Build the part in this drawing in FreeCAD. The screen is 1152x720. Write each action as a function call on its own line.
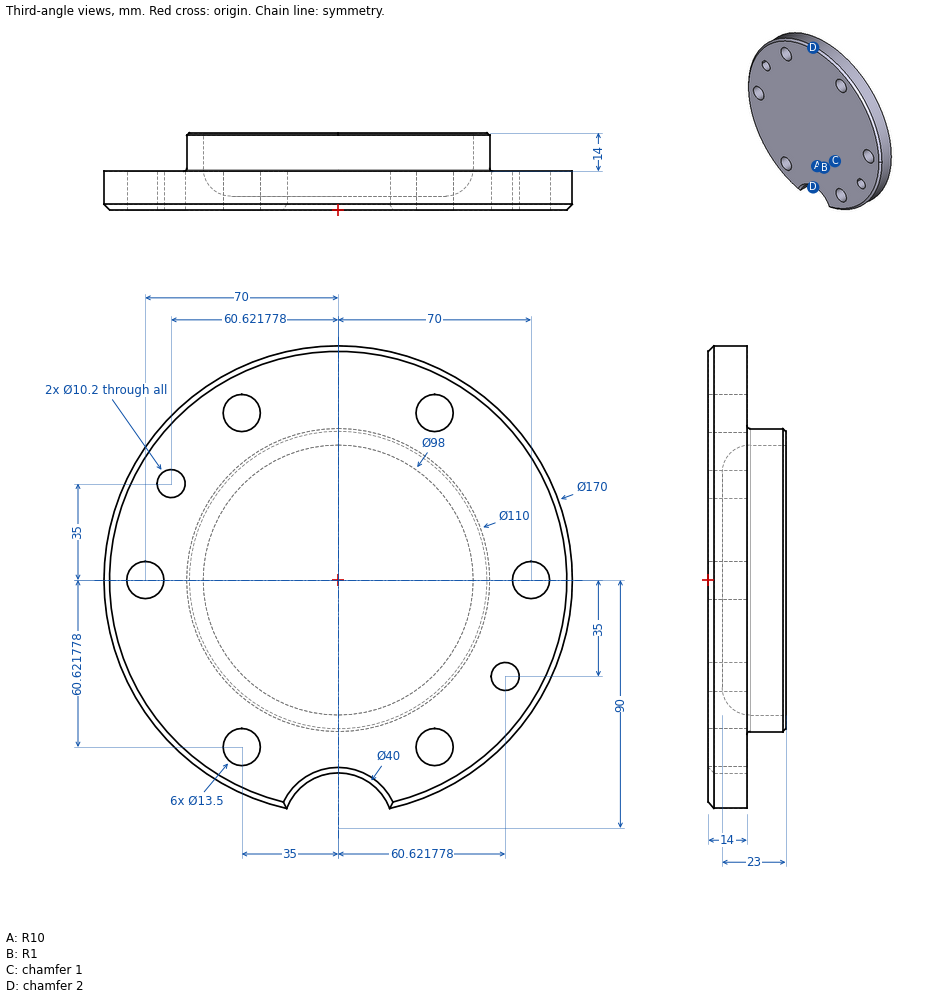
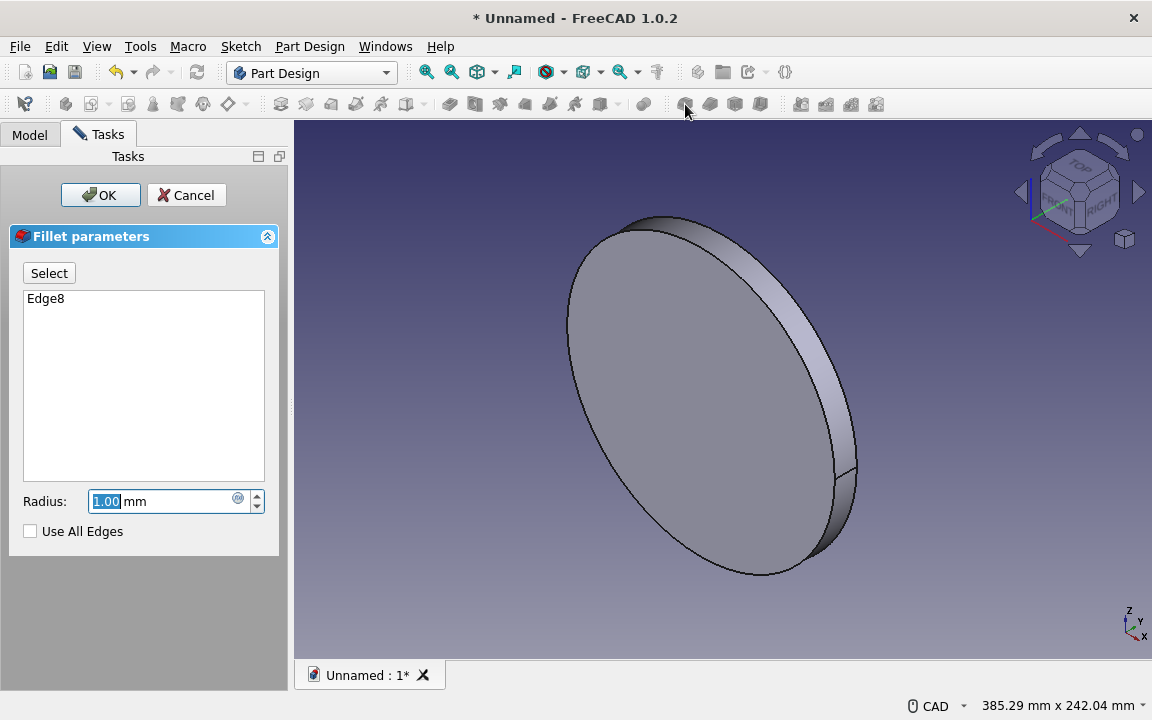
text(1)
key(Tab)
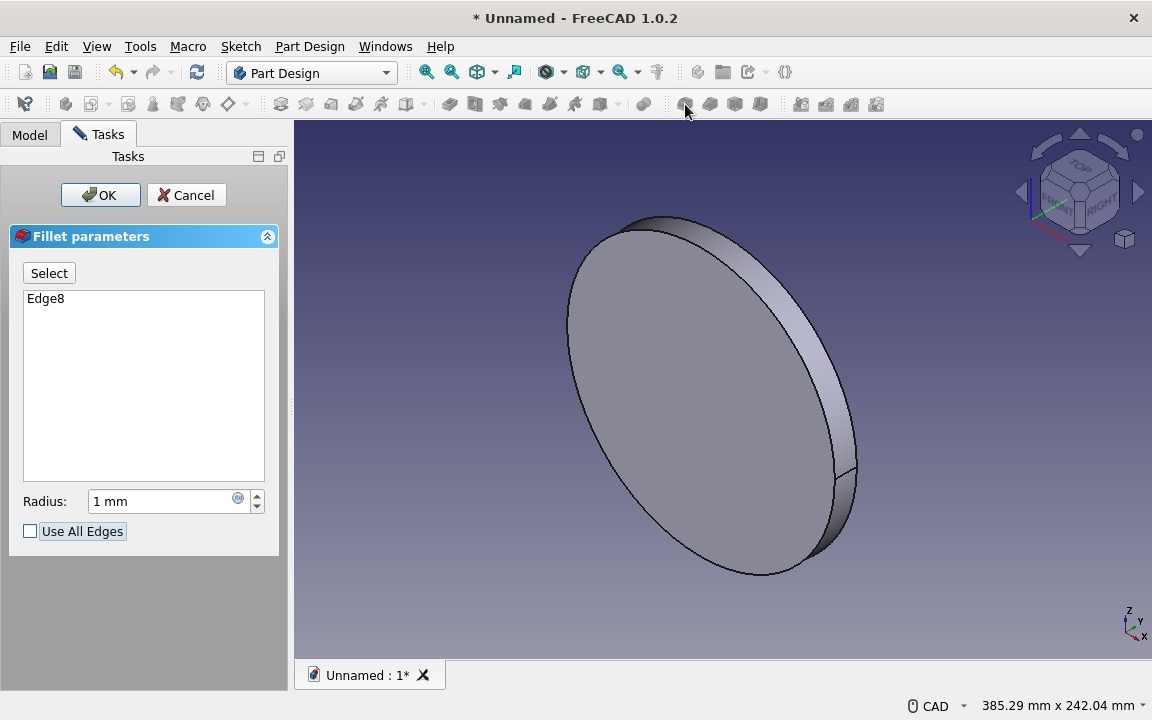
click(101, 195)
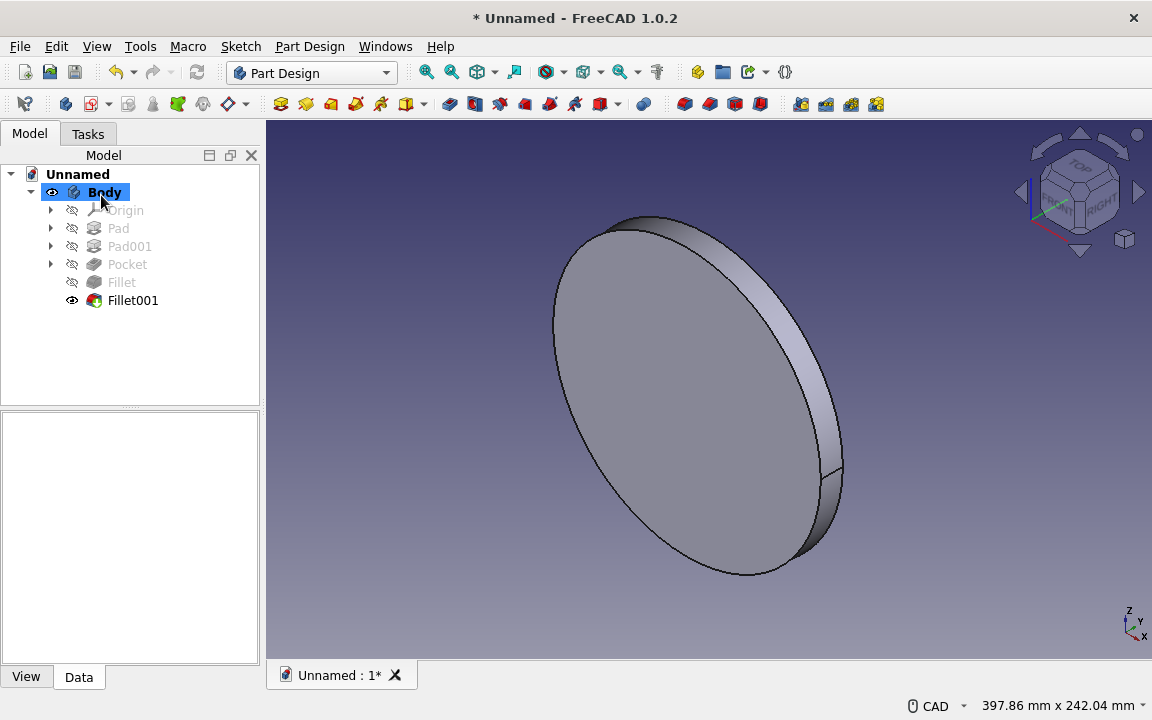
key(2)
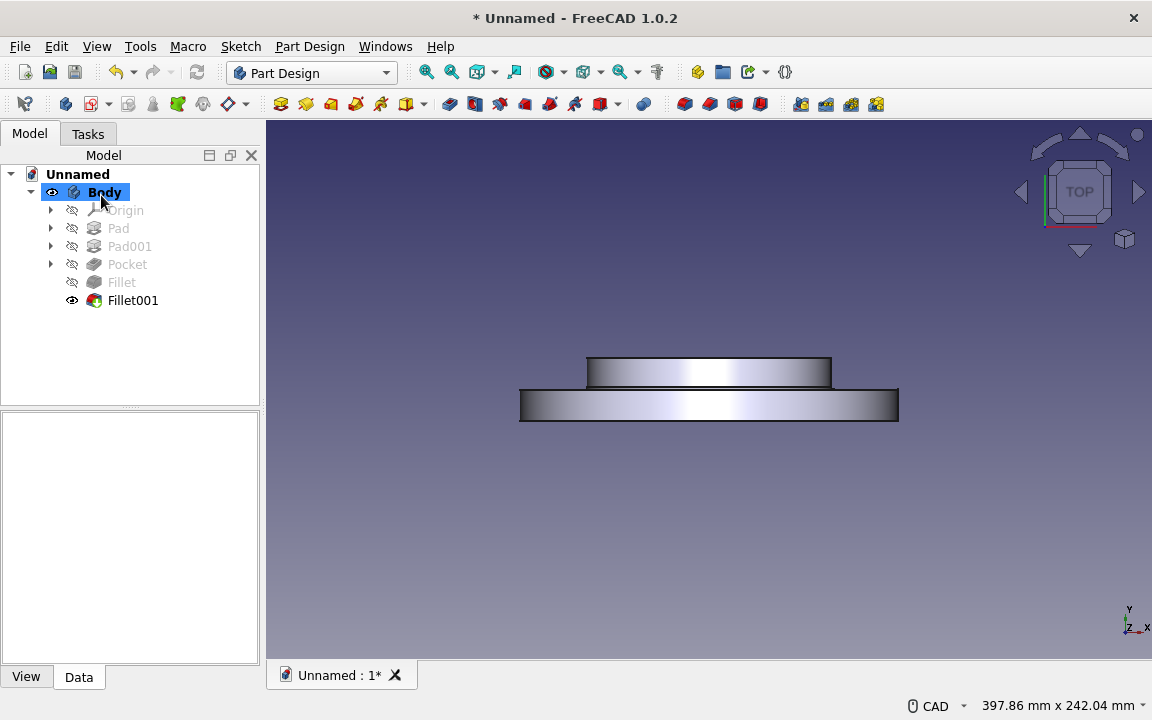
click(427, 72)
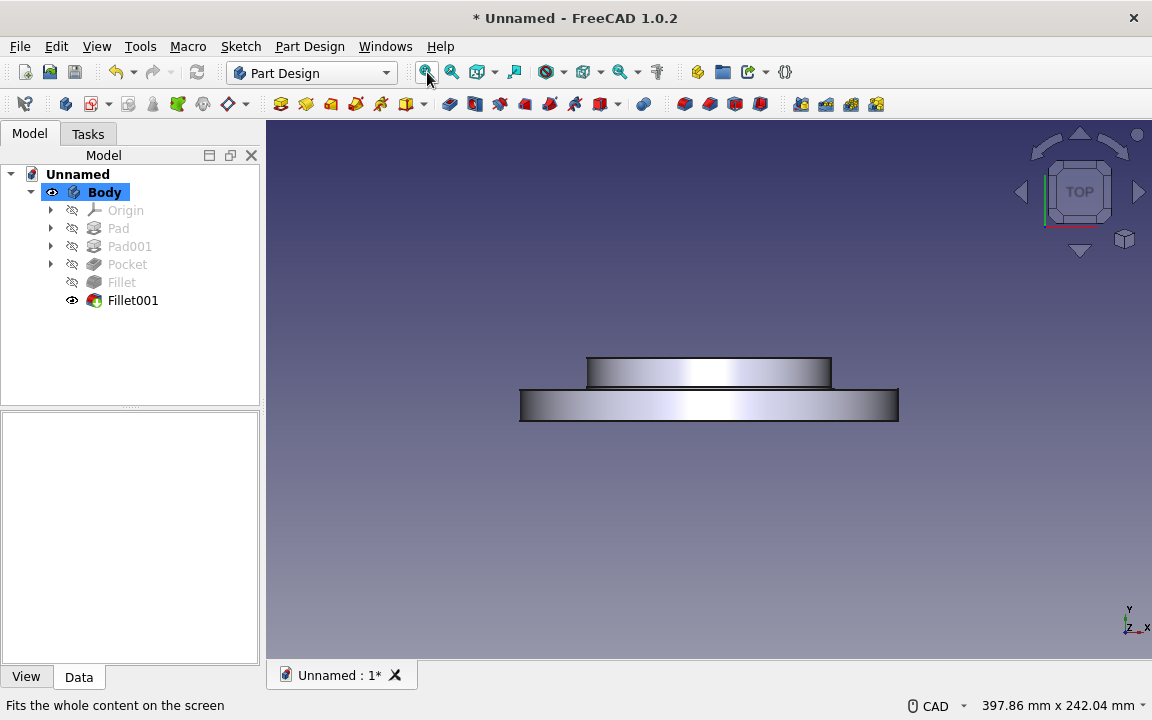
click(610, 357)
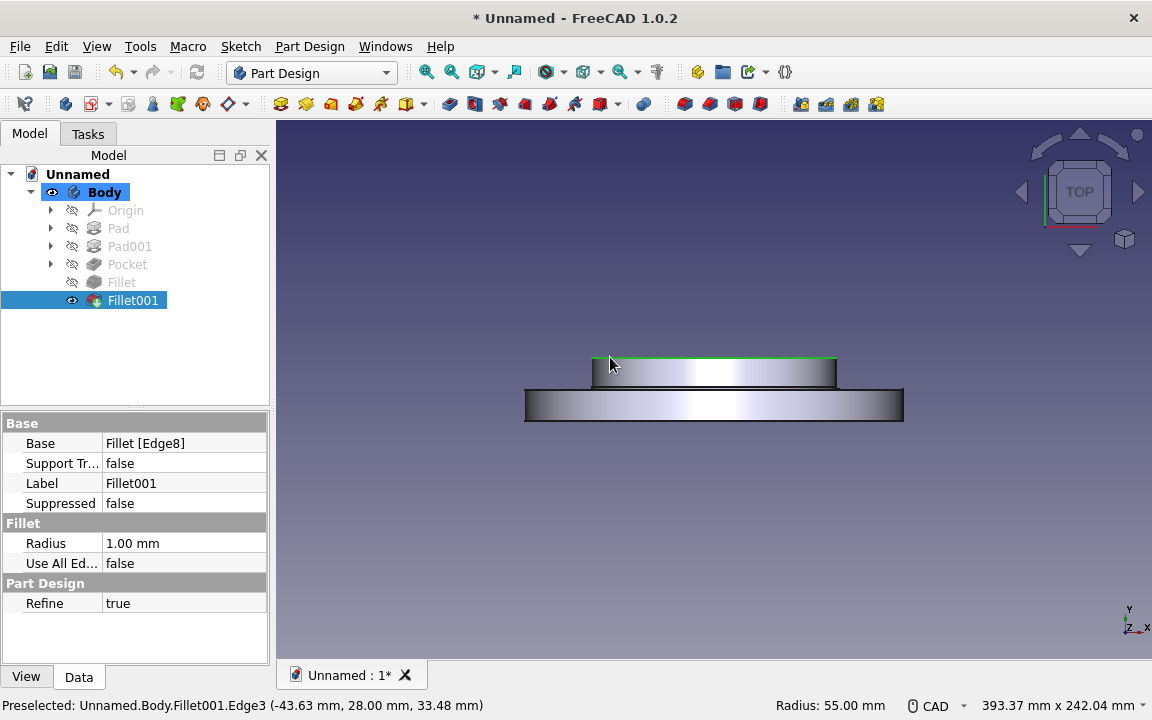
click(710, 104)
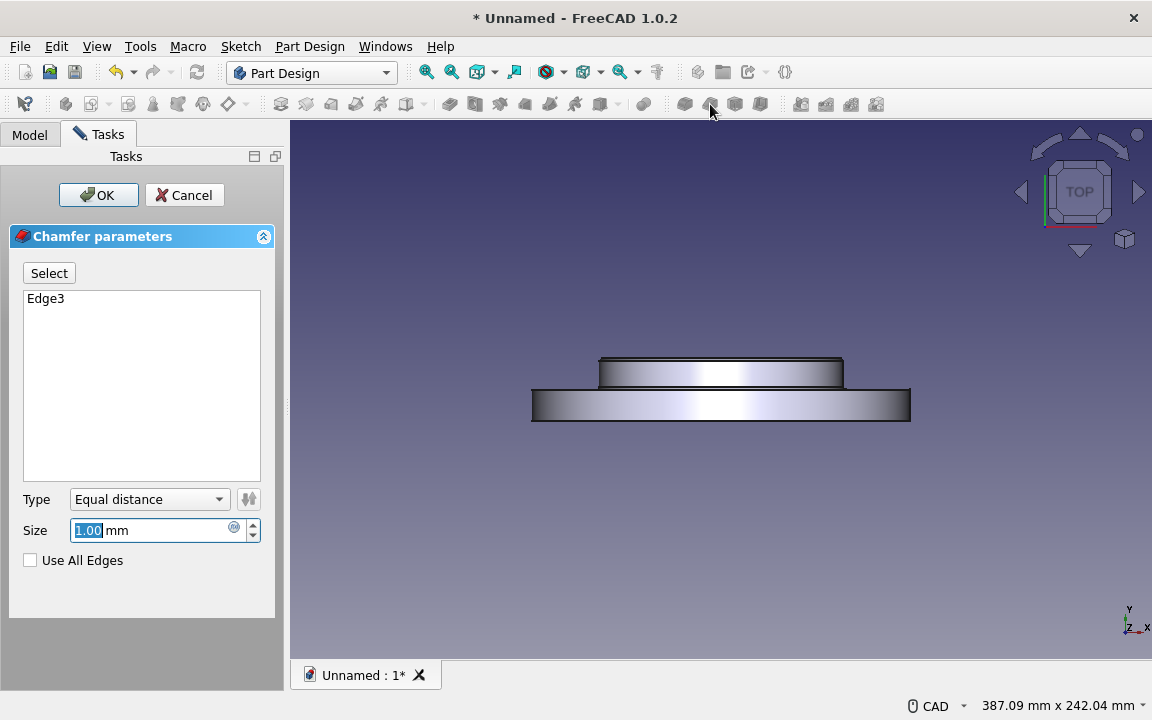
text(1)
key(Tab)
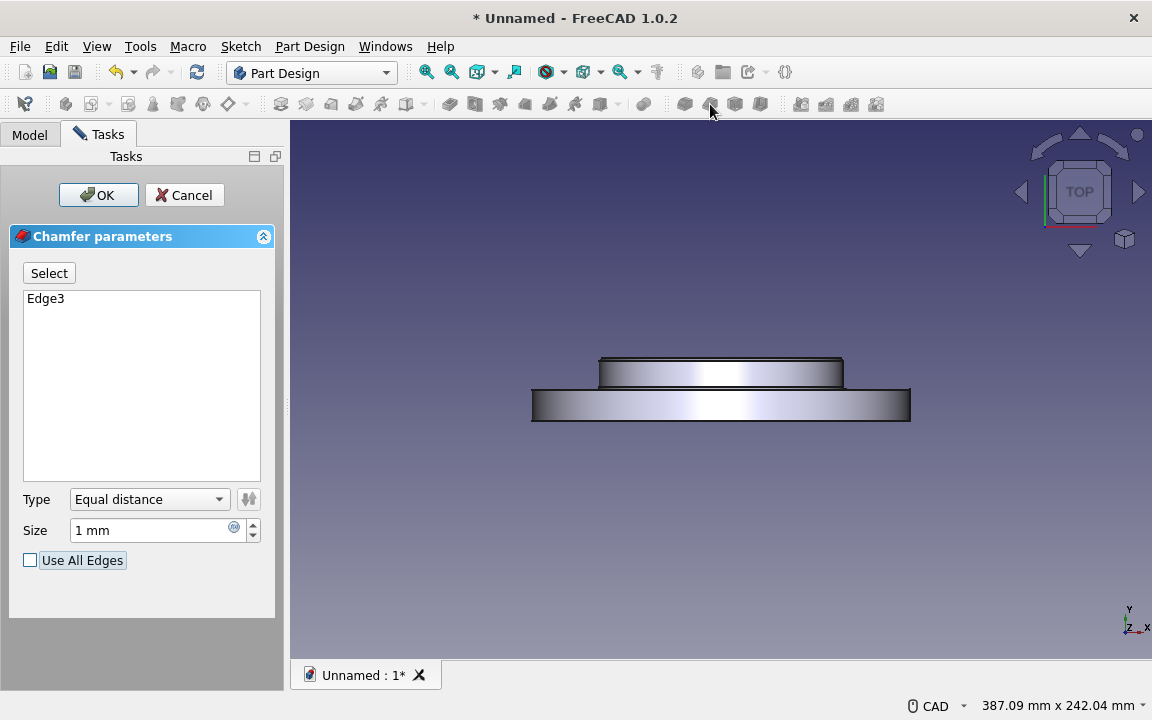
click(99, 195)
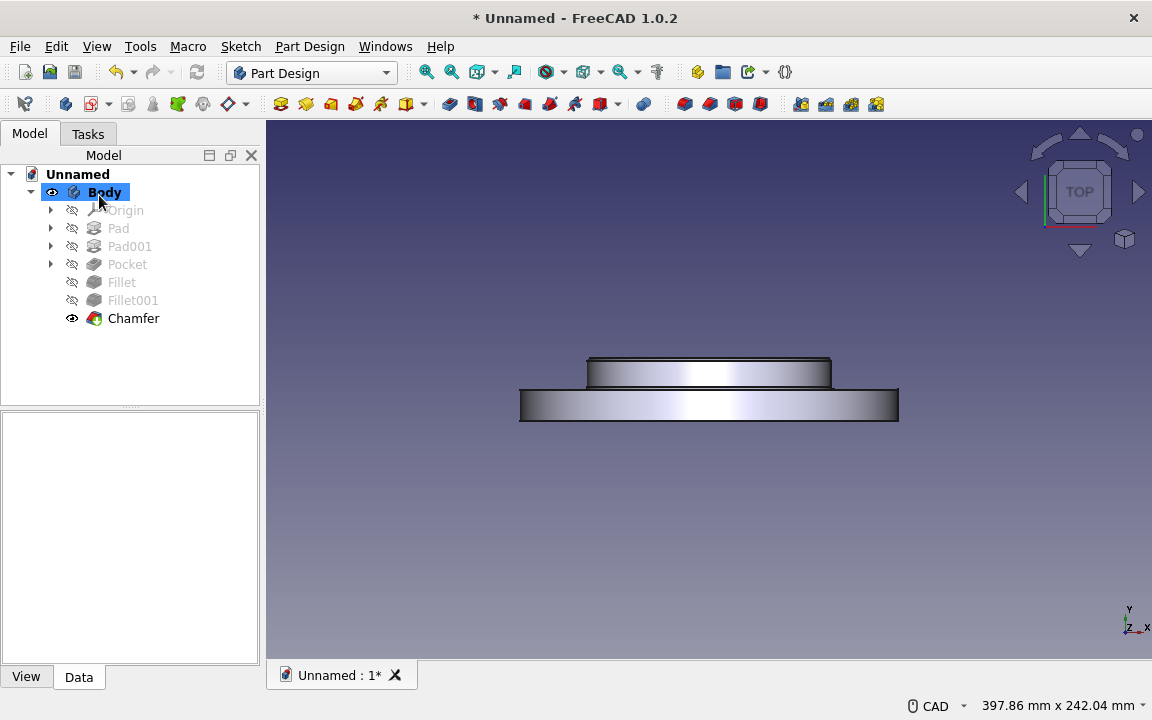
click(427, 72)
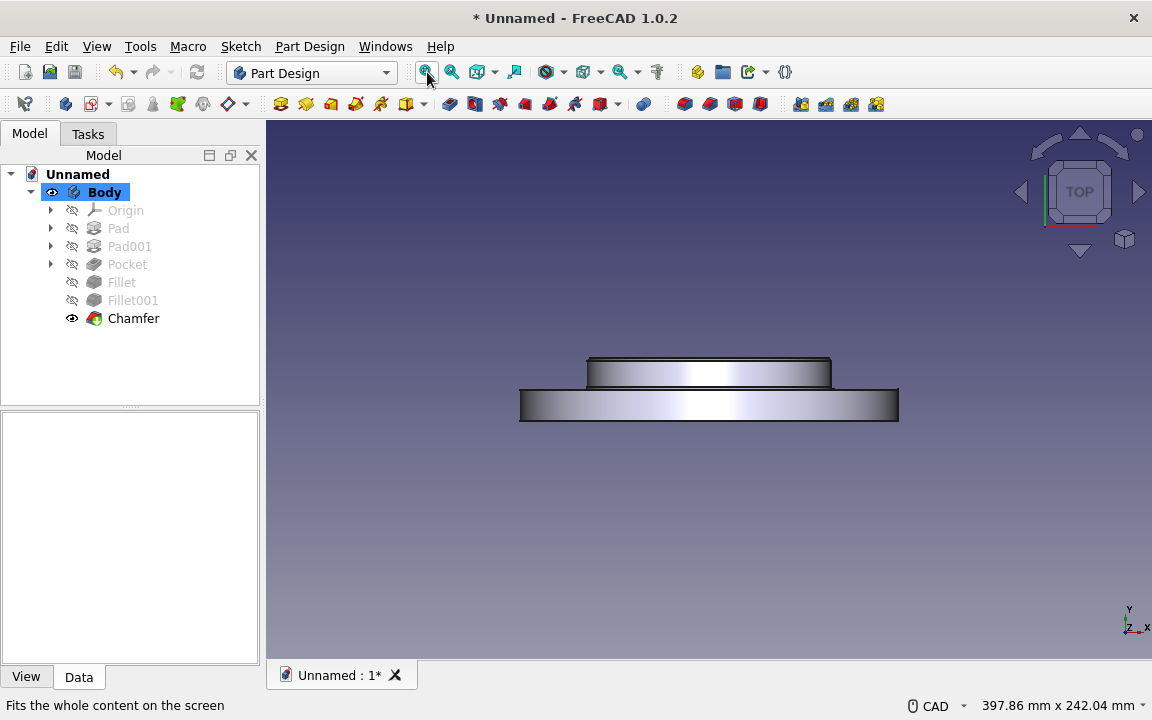
key(4)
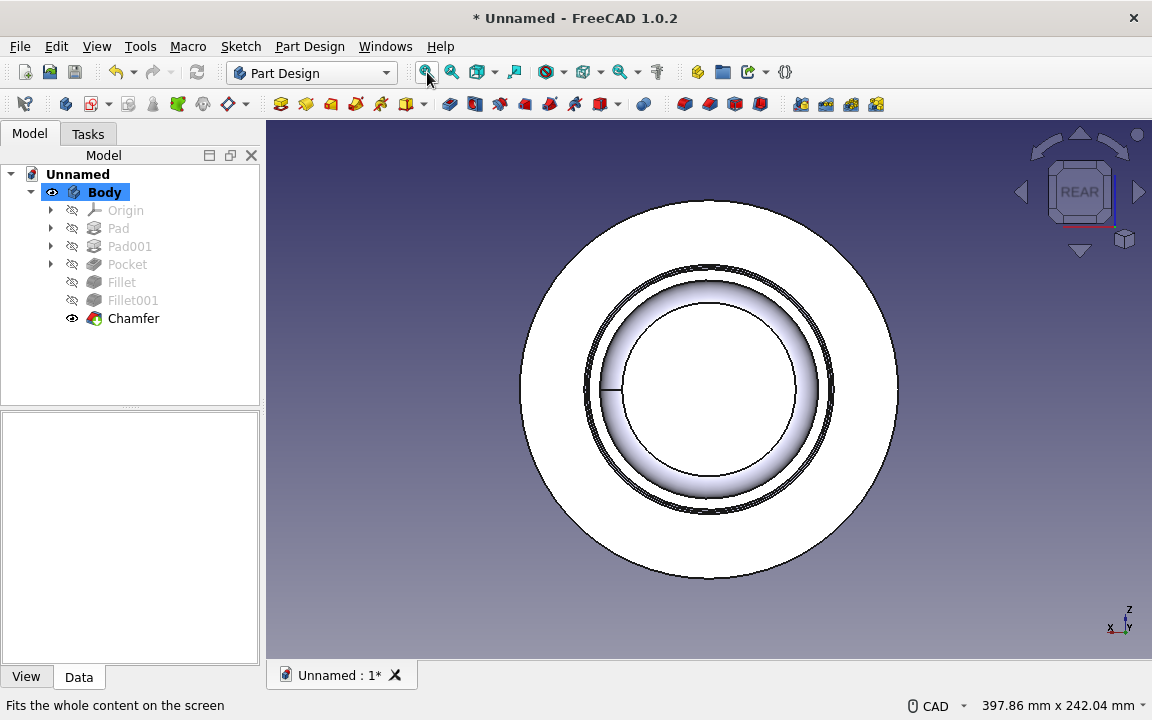
click(601, 280)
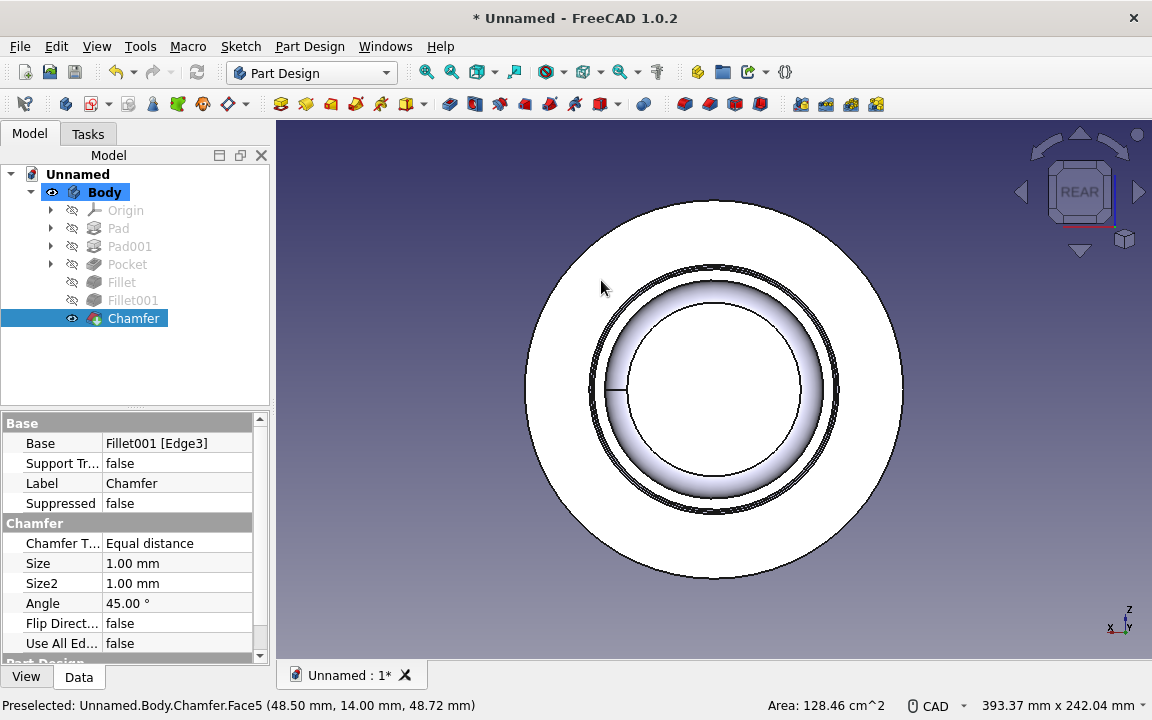
click(90, 104)